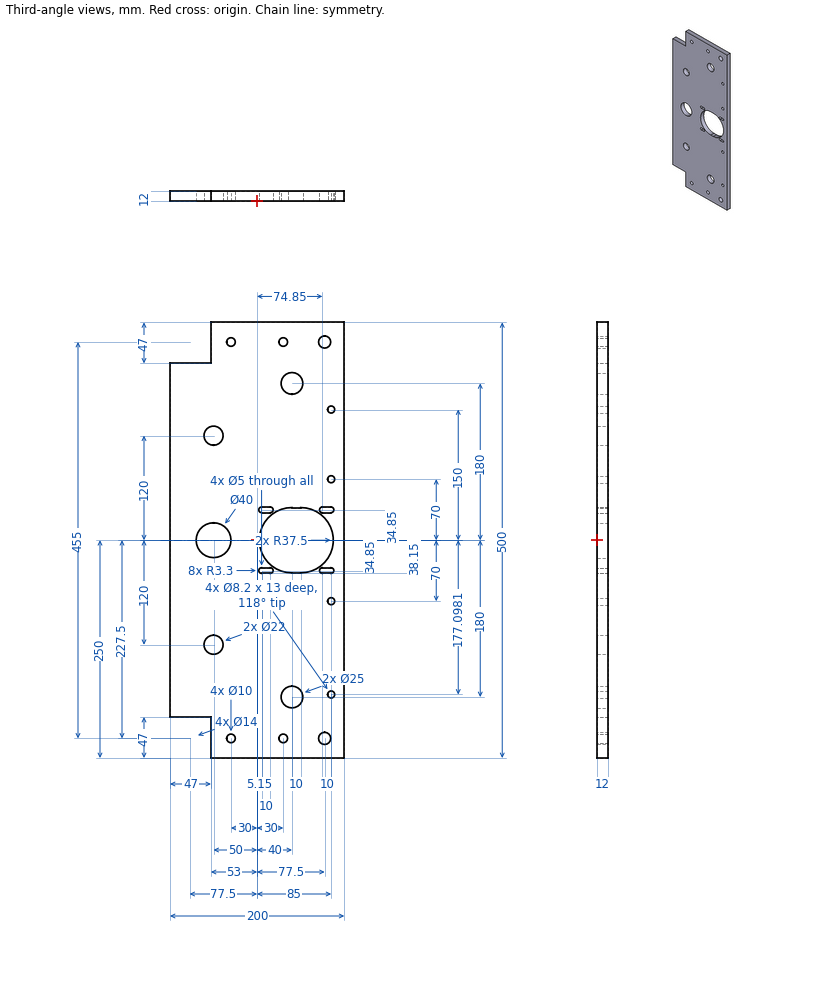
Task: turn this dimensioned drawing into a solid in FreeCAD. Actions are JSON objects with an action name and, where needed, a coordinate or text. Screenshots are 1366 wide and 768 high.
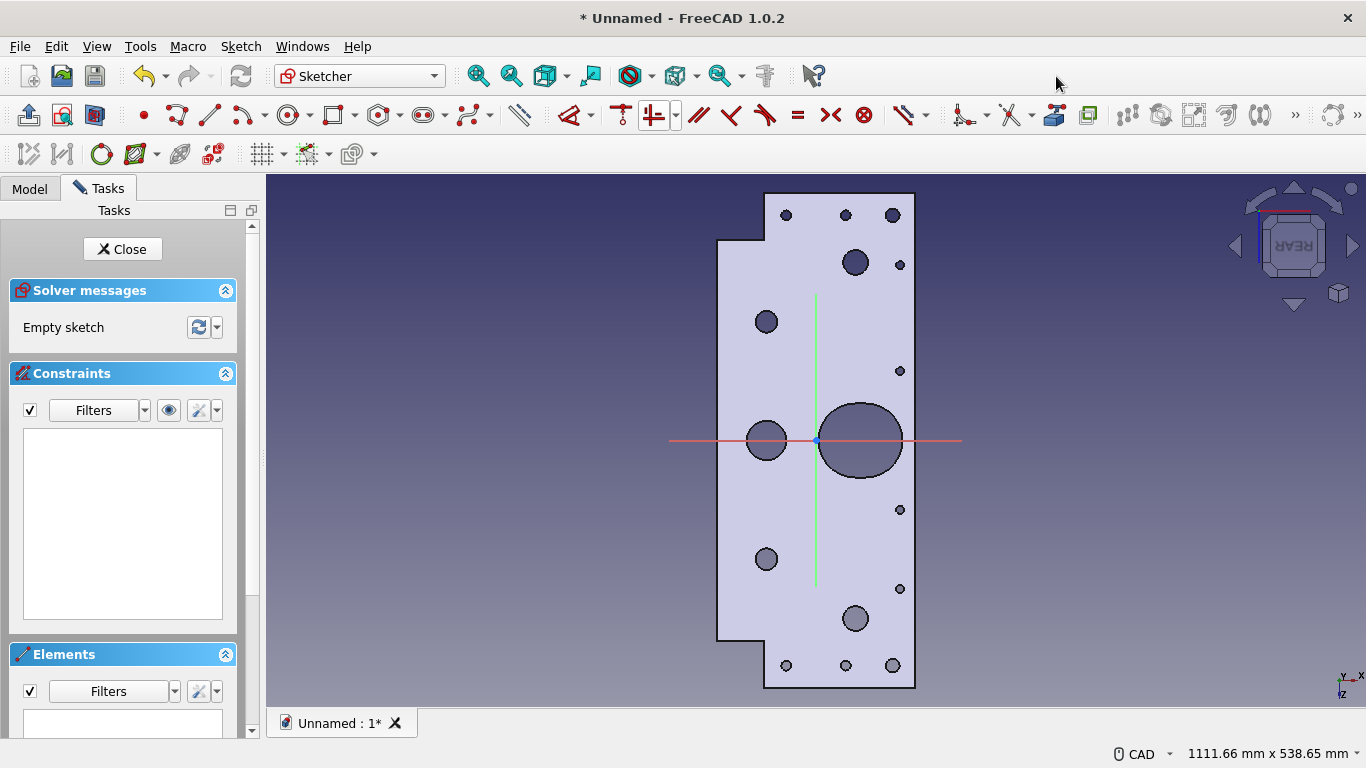
{"action": "scroll", "coordinate": [881, 440], "scroll_direction": "up", "scroll_amount": 8}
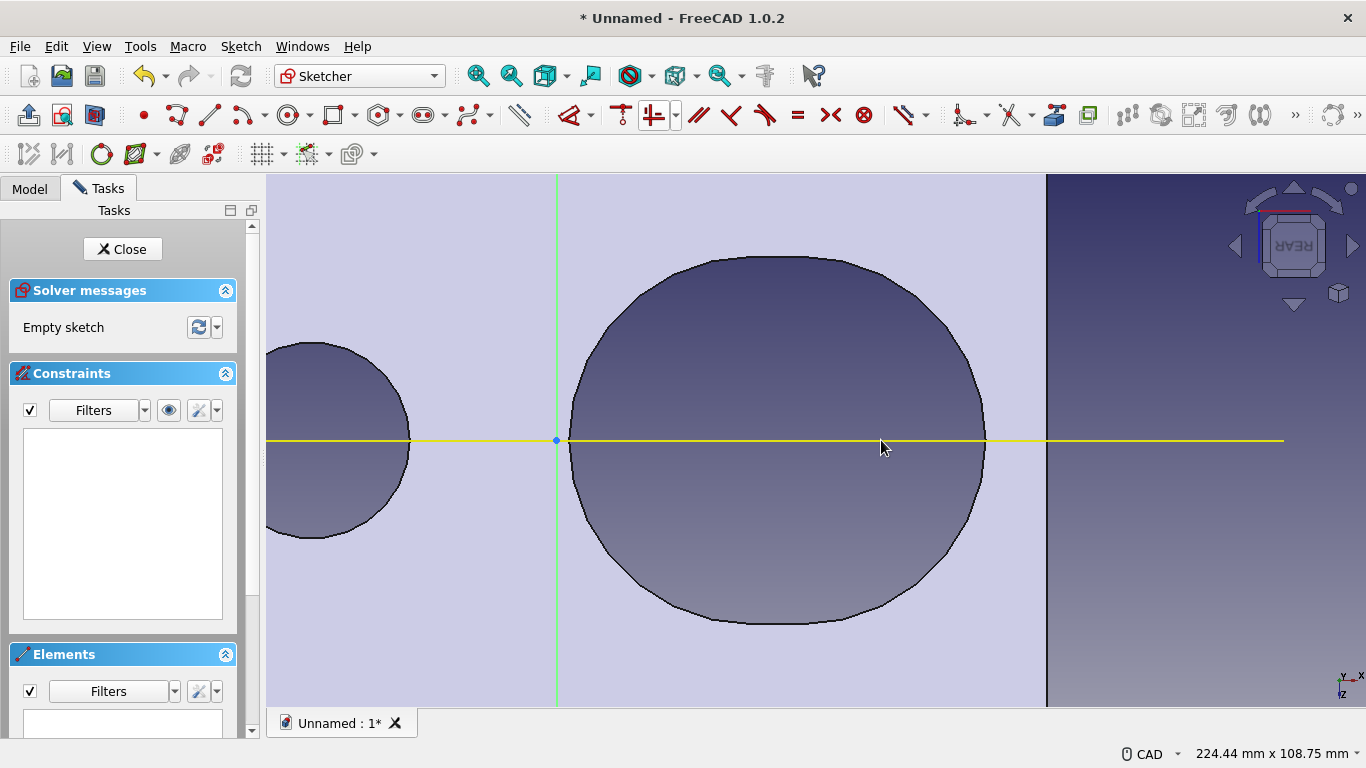
{"action": "key", "text": "g c"}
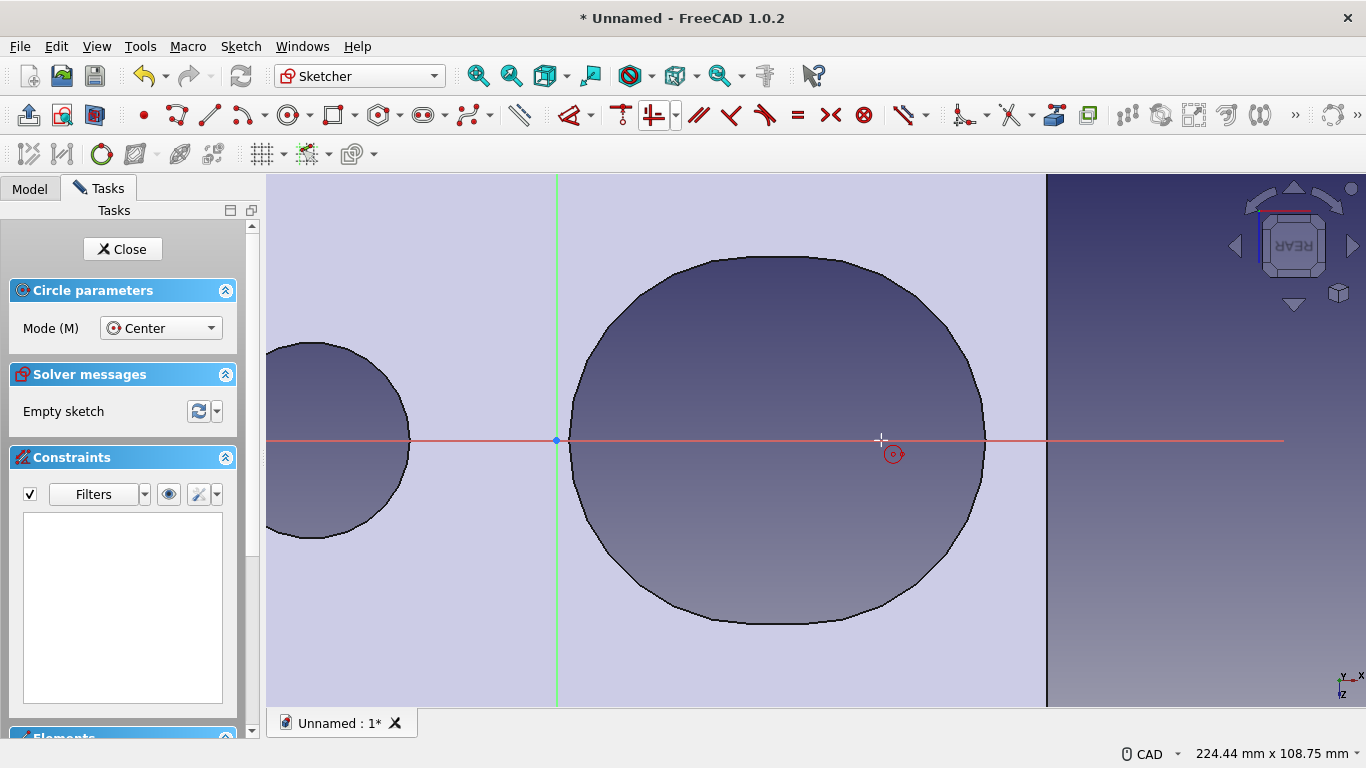
{"action": "scroll", "coordinate": [582, 270], "scroll_direction": "up", "scroll_amount": 4}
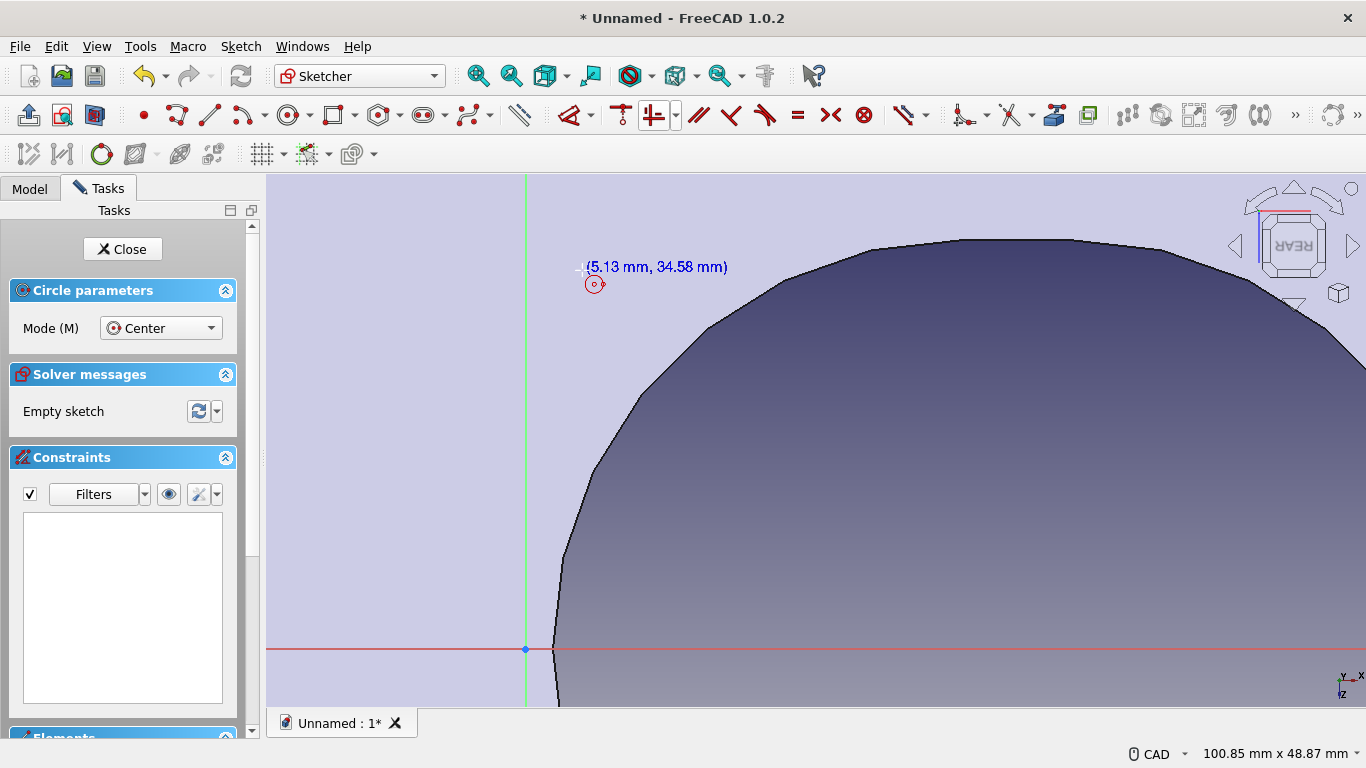
{"action": "left_click", "coordinate": [582, 269]}
{"action": "mouse_move", "coordinate": [601, 250]}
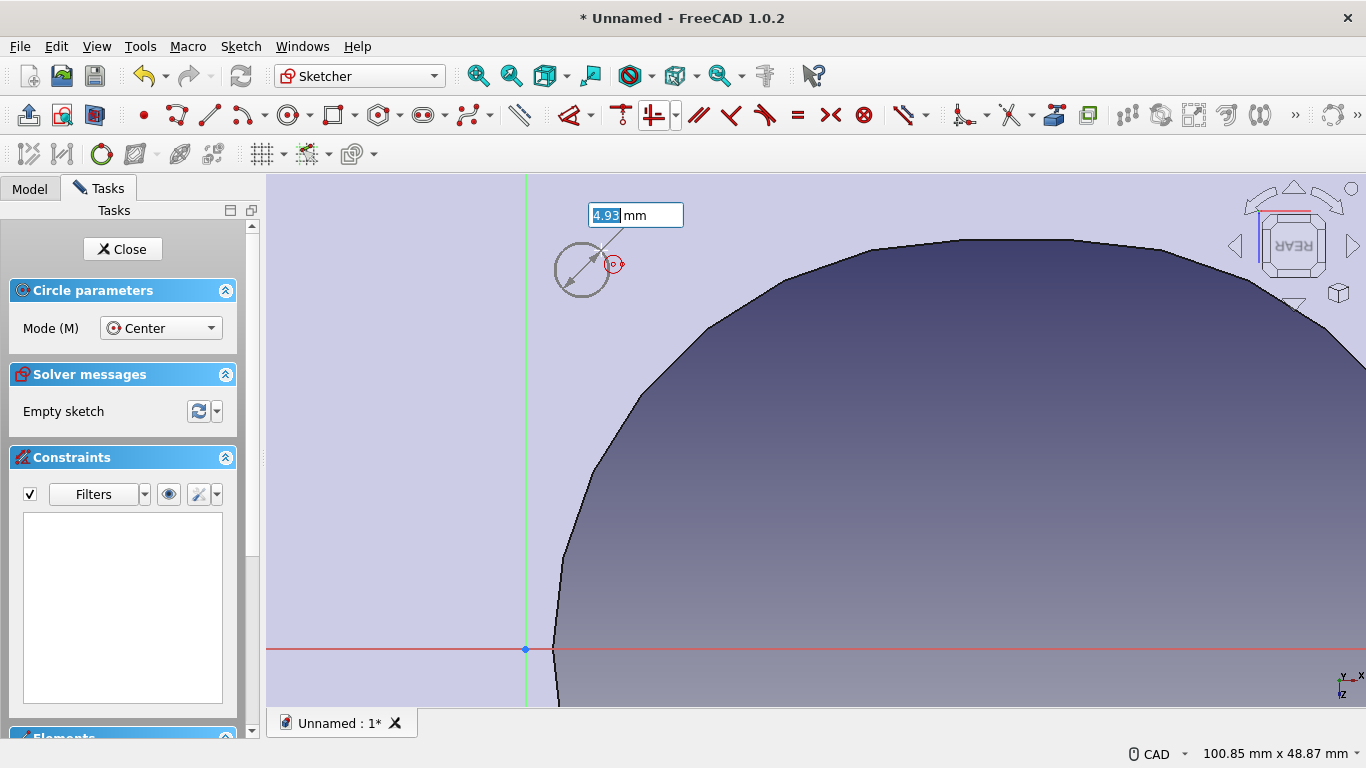
{"action": "type", "text": "5"}
{"action": "key", "text": "Return"}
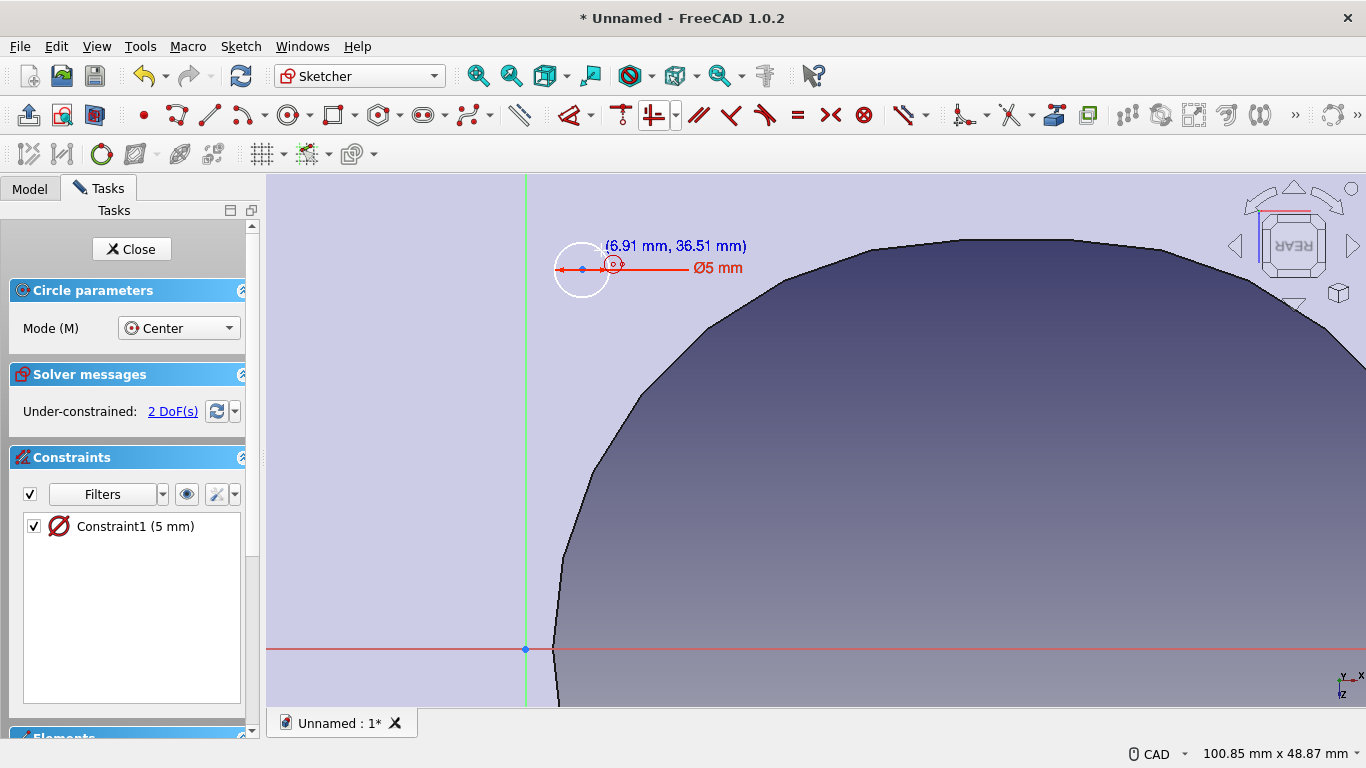
{"action": "scroll", "coordinate": [584, 270], "scroll_direction": "down", "scroll_amount": 4}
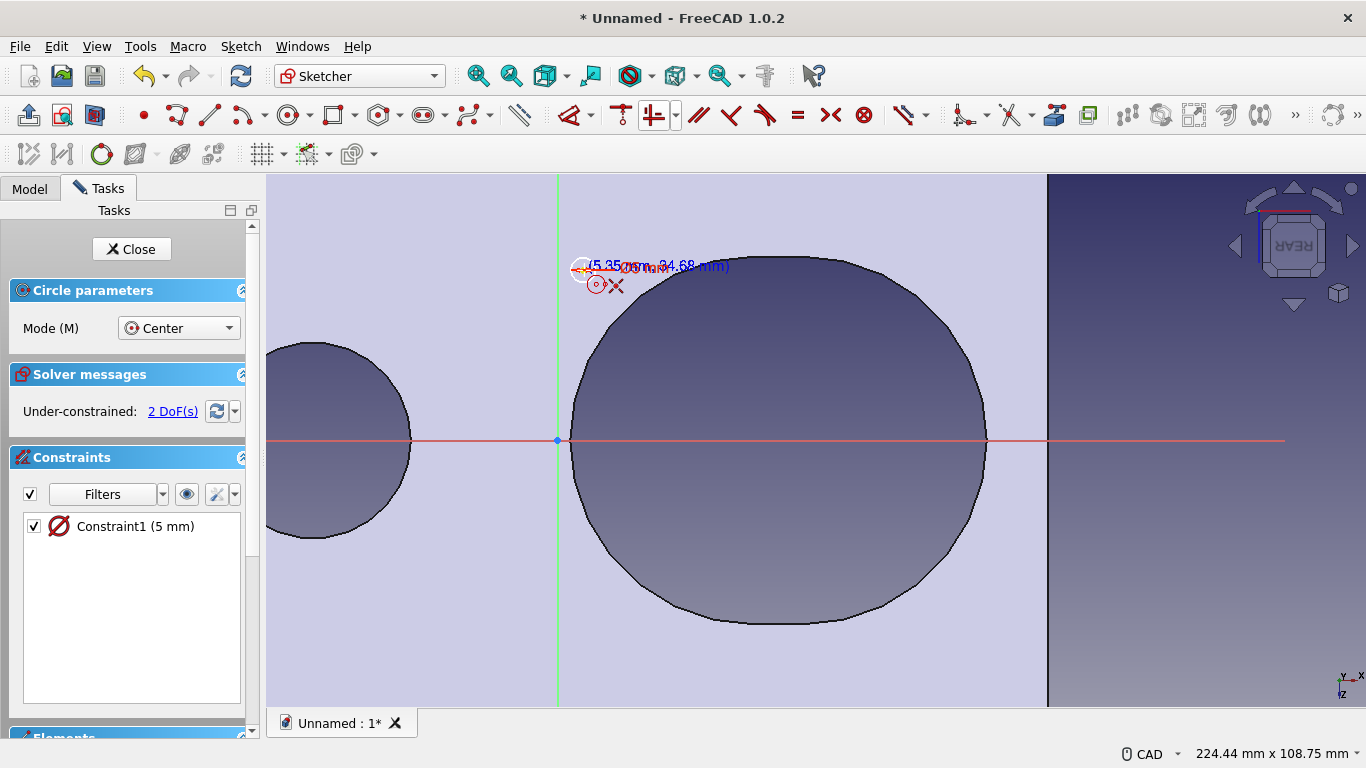
{"action": "scroll", "coordinate": [583, 611], "scroll_direction": "up", "scroll_amount": 4}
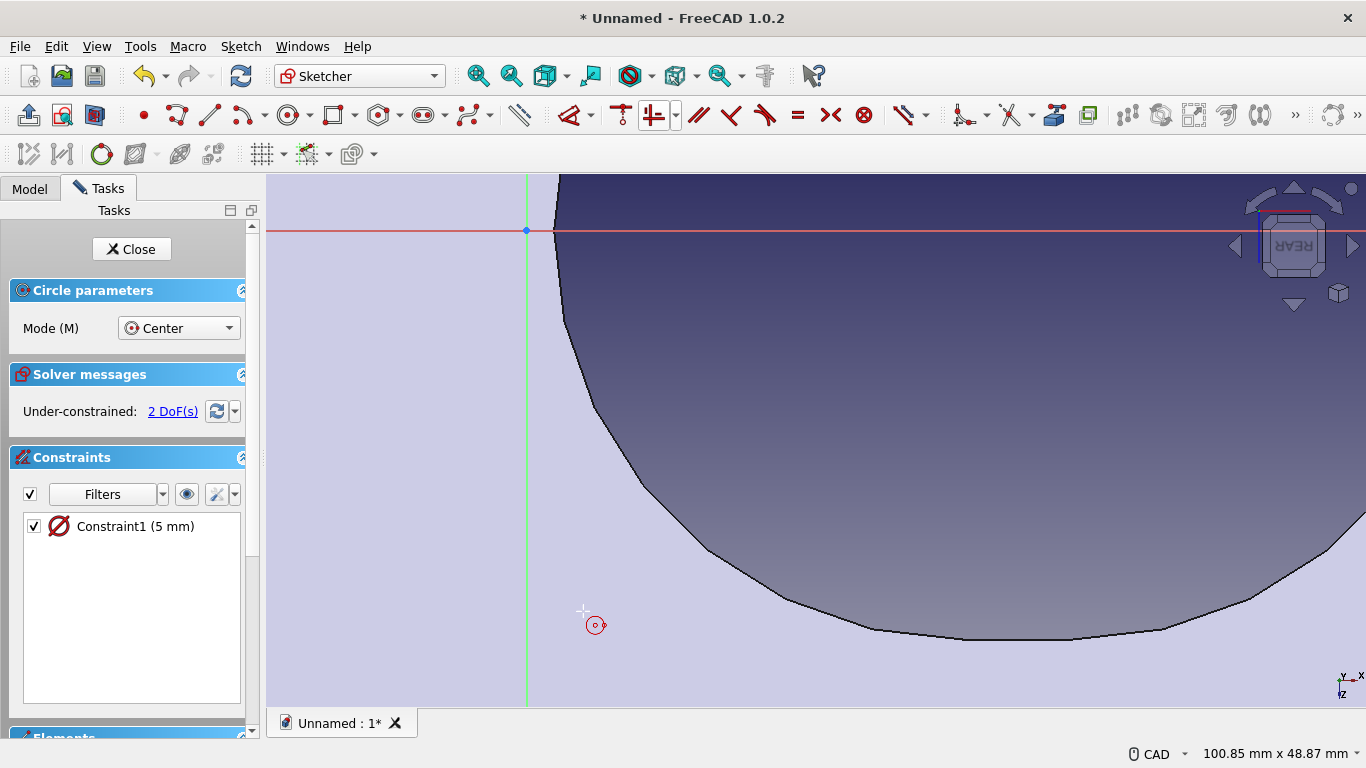
{"action": "left_click", "coordinate": [583, 611]}
{"action": "mouse_move", "coordinate": [602, 591]}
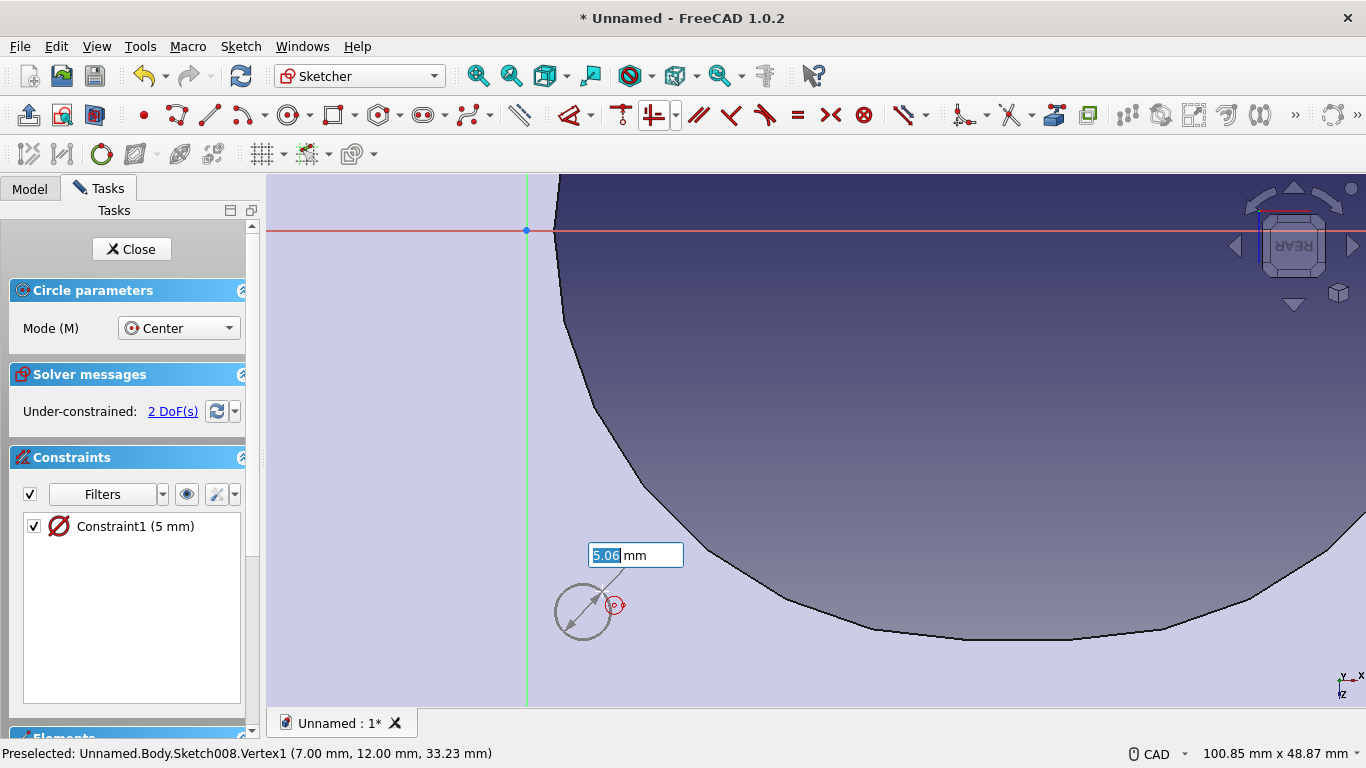
{"action": "type", "text": "5"}
{"action": "key", "text": "Return"}